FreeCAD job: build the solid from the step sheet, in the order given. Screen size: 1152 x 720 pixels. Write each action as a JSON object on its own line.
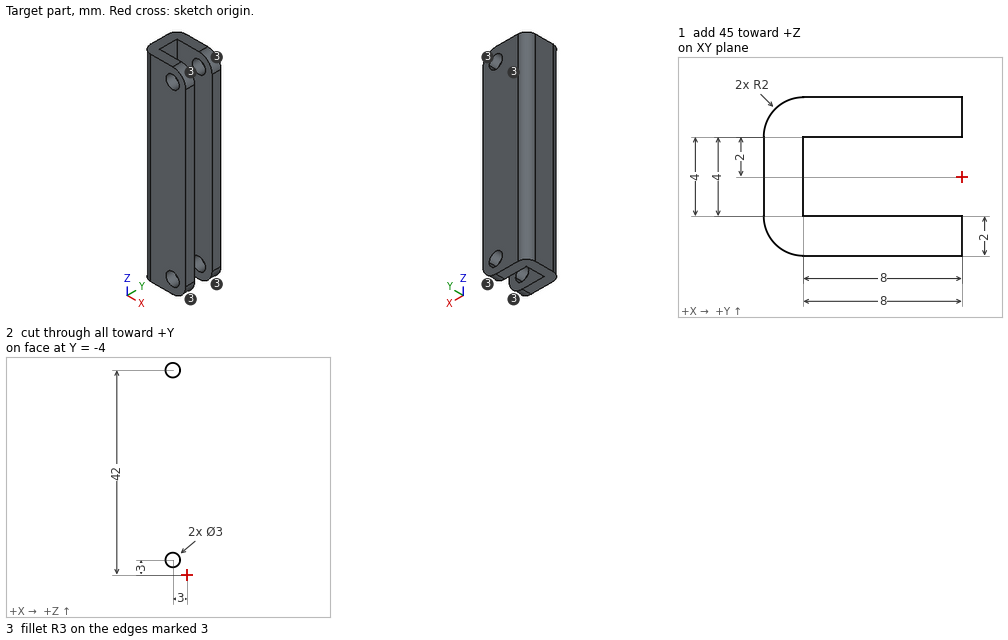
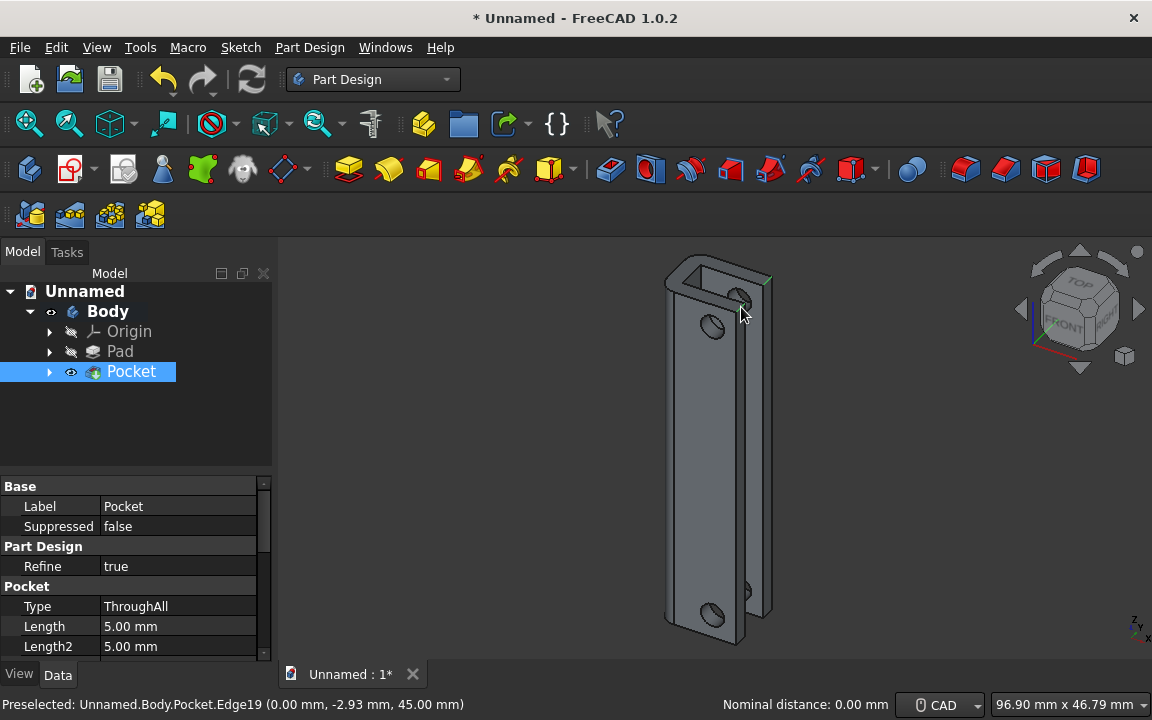
{"action": "scroll", "coordinate": [768, 613], "scroll_direction": "up", "scroll_amount": 4}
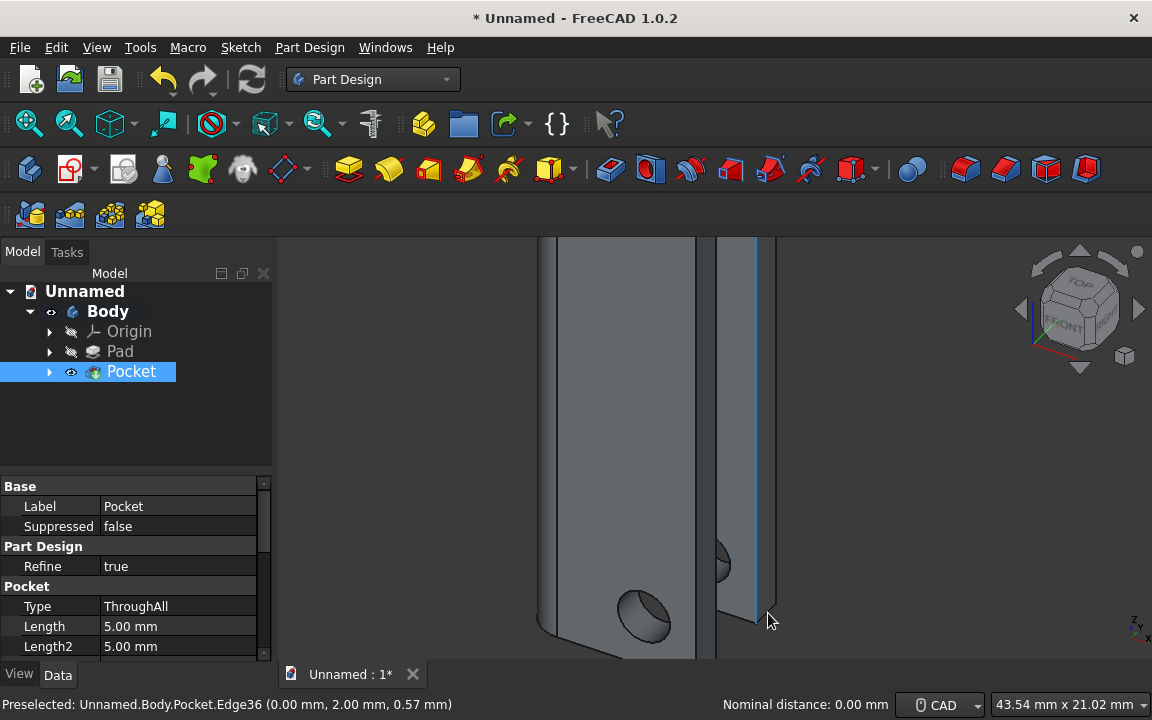
{"action": "left_click", "coordinate": [30, 124]}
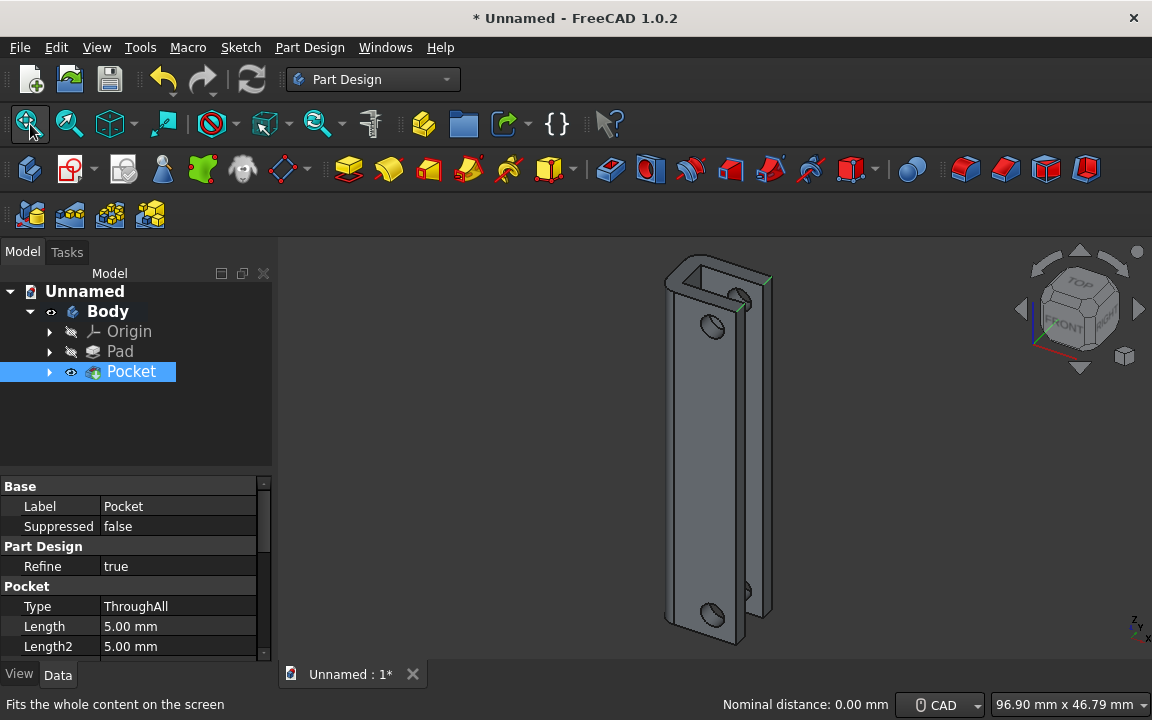
{"action": "key", "text": "0"}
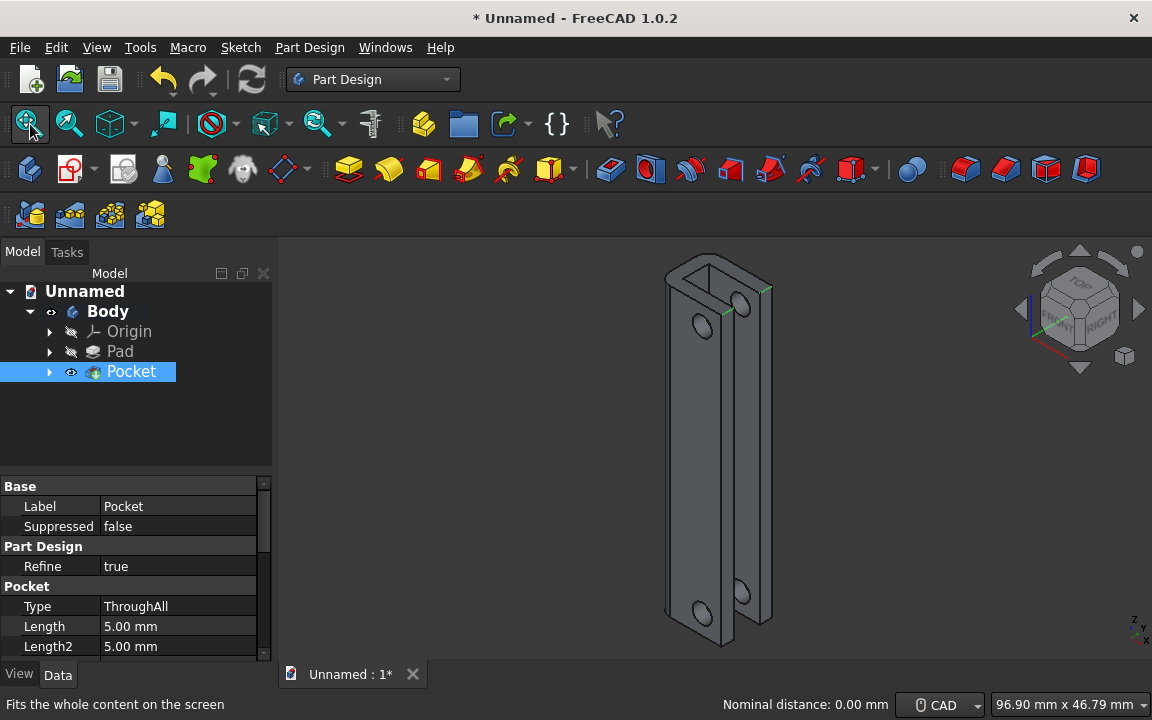
{"action": "scroll", "coordinate": [766, 620], "scroll_direction": "up", "scroll_amount": 4}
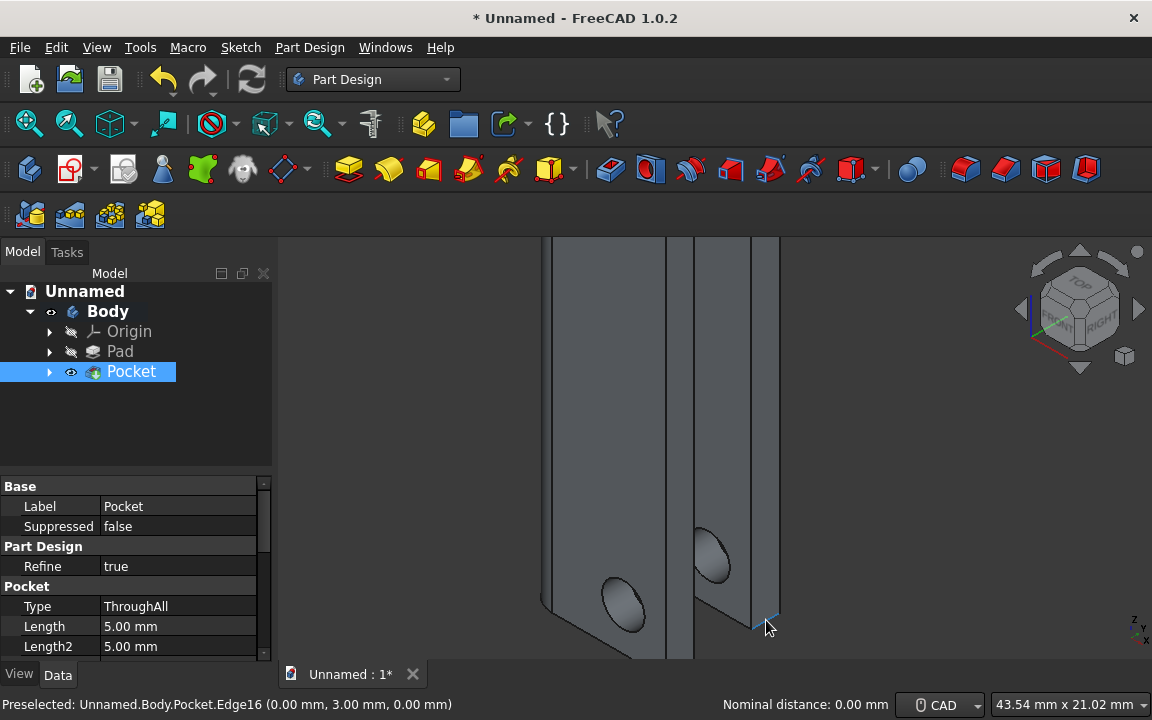
{"action": "left_click", "coordinate": [30, 124]}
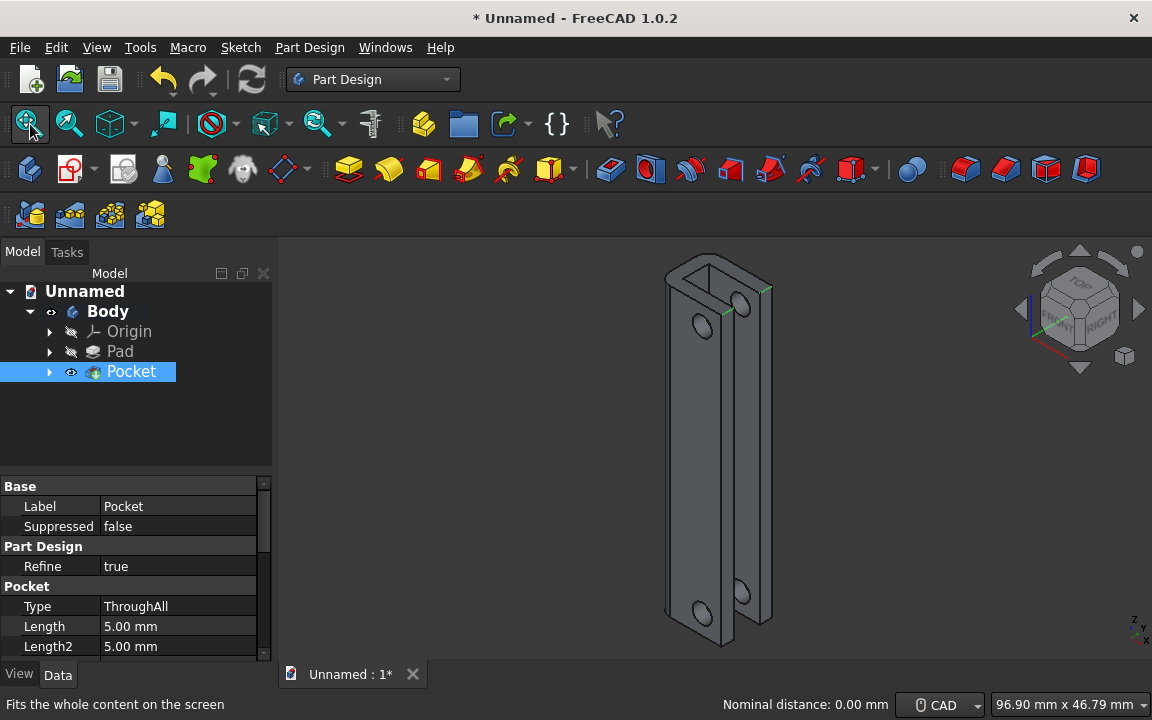
{"action": "key", "text": "2"}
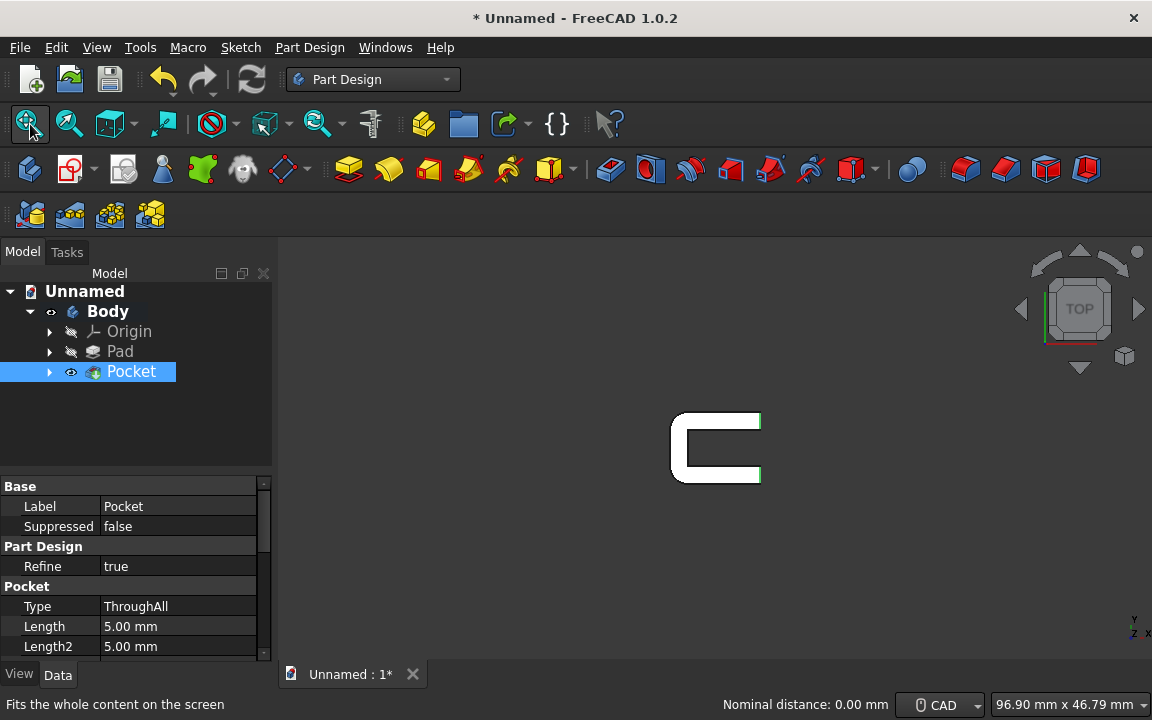
{"action": "left_click", "coordinate": [30, 124]}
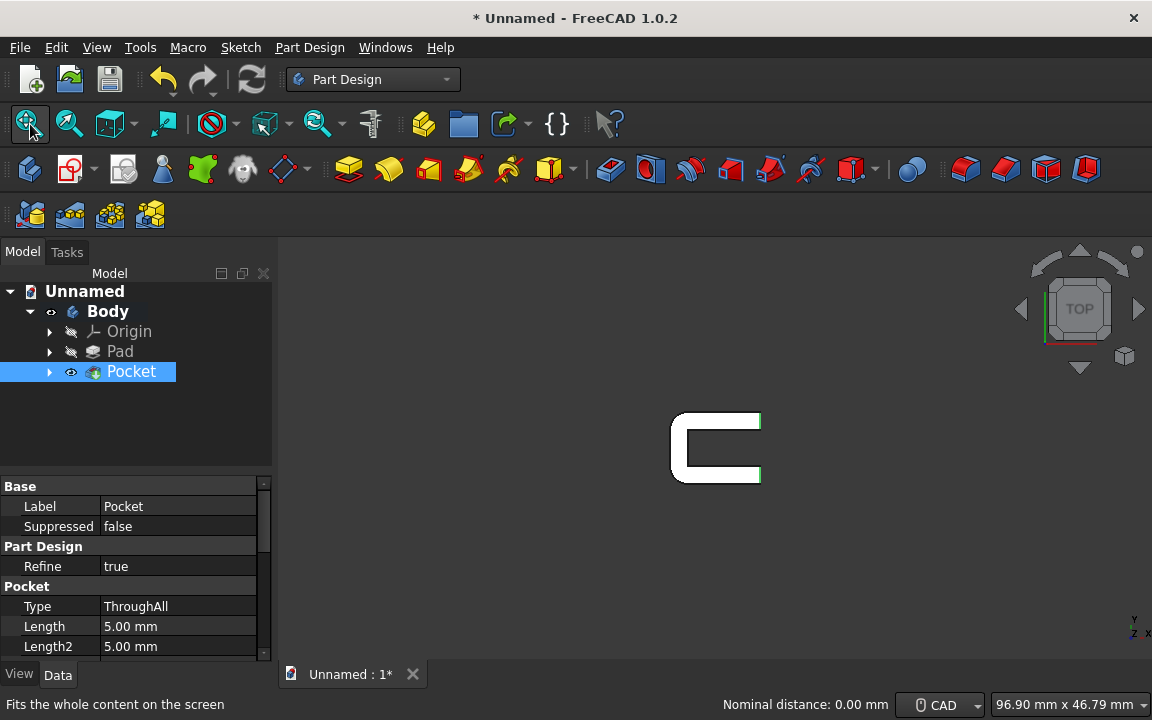
{"action": "scroll", "coordinate": [760, 420], "scroll_direction": "up", "scroll_amount": 4}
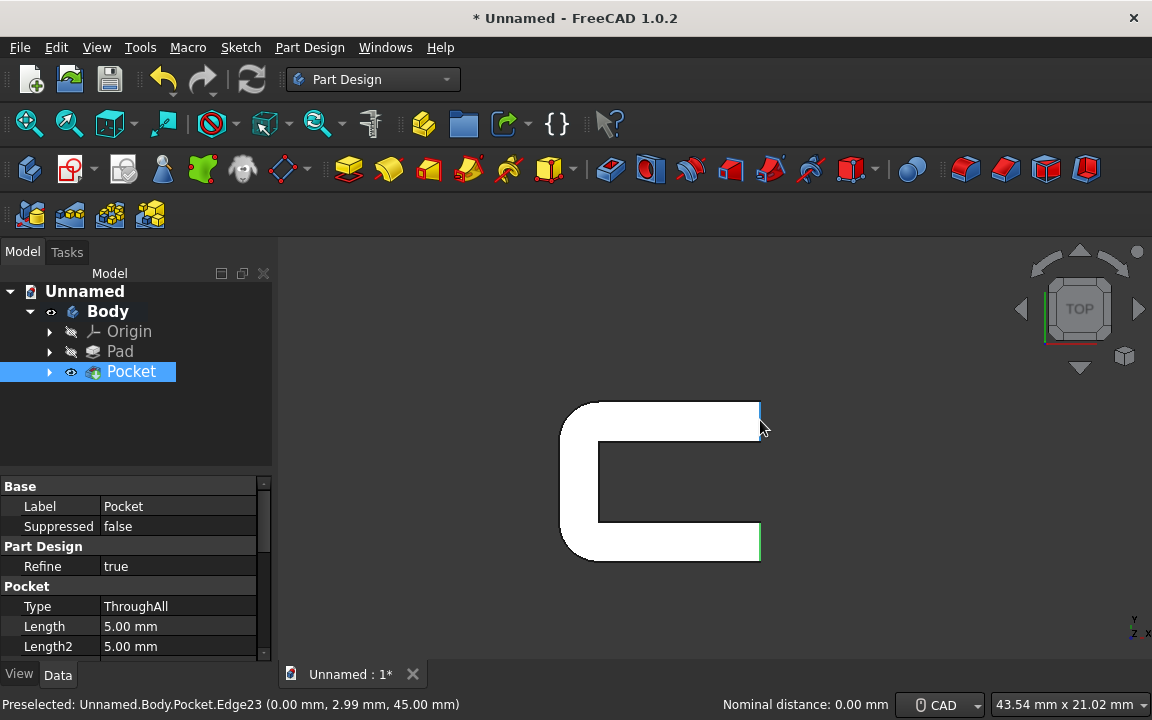
{"action": "left_click", "coordinate": [30, 124]}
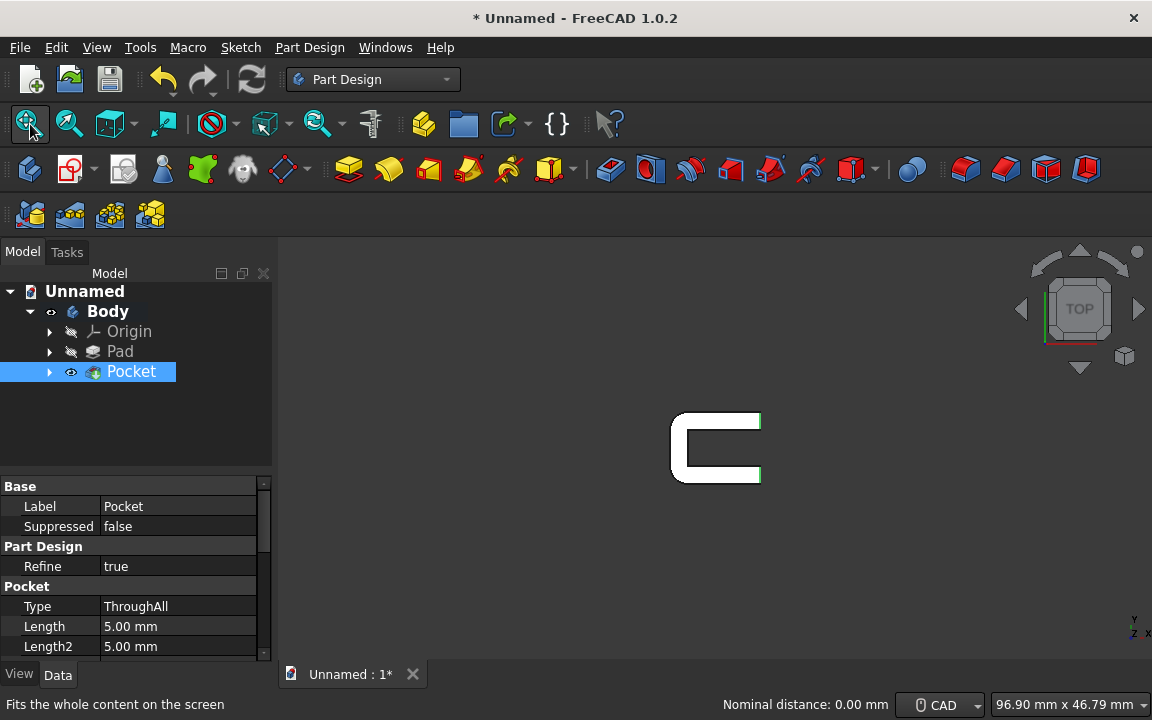
{"action": "key", "text": "1"}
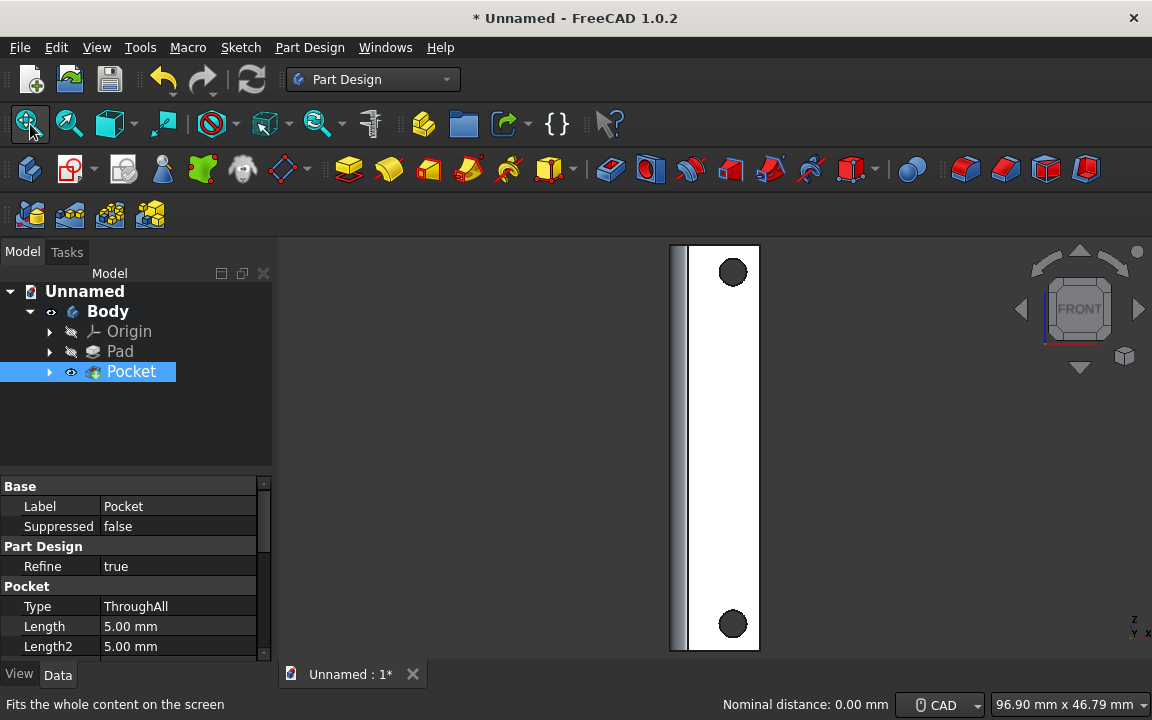
{"action": "key", "text": "3"}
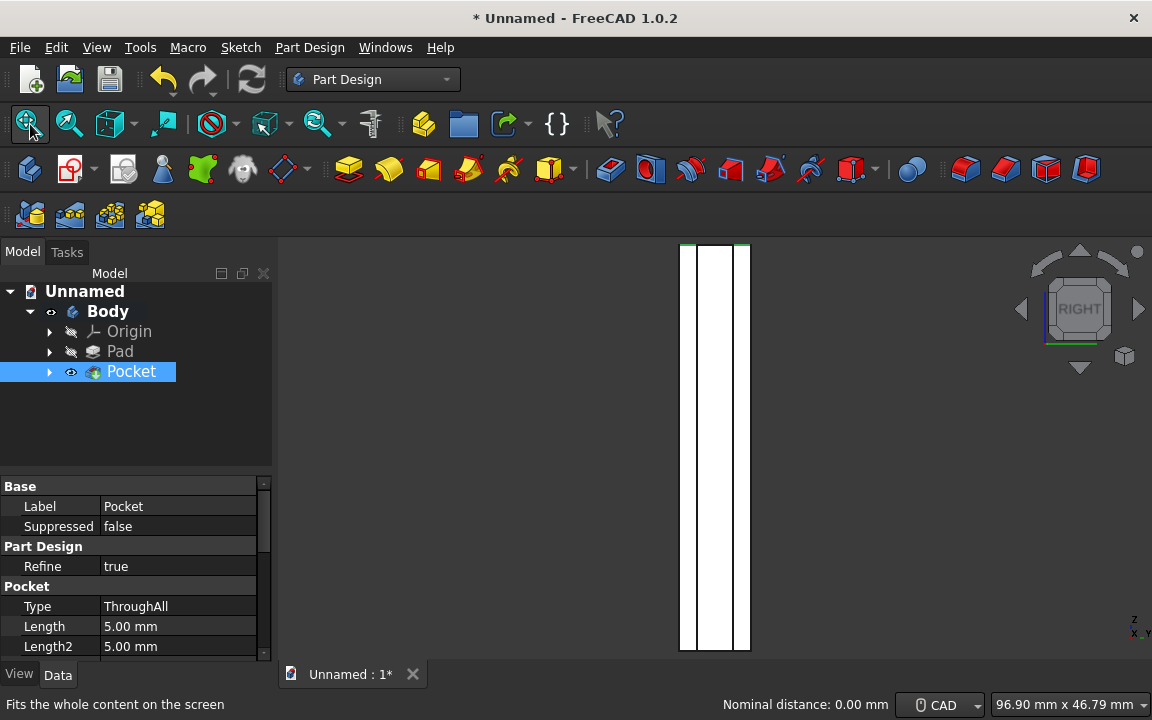
{"action": "key", "text": "5"}